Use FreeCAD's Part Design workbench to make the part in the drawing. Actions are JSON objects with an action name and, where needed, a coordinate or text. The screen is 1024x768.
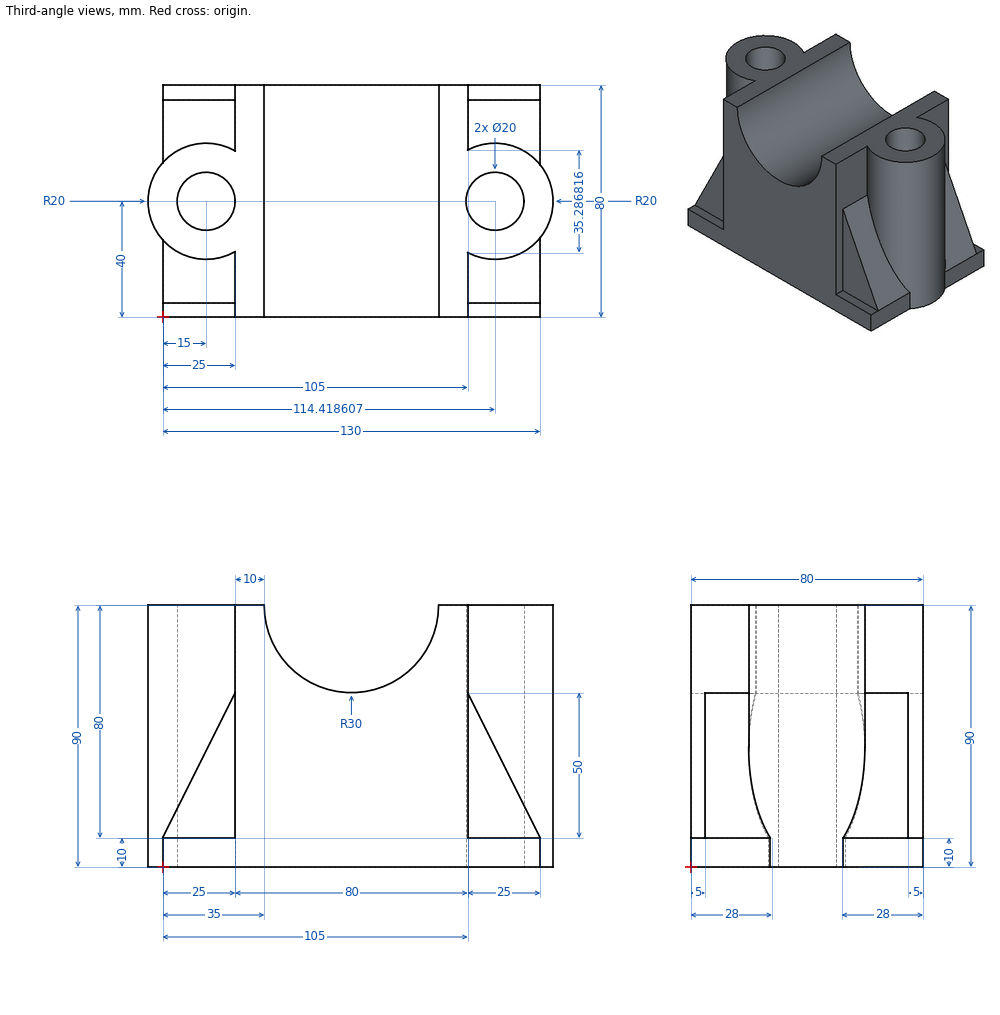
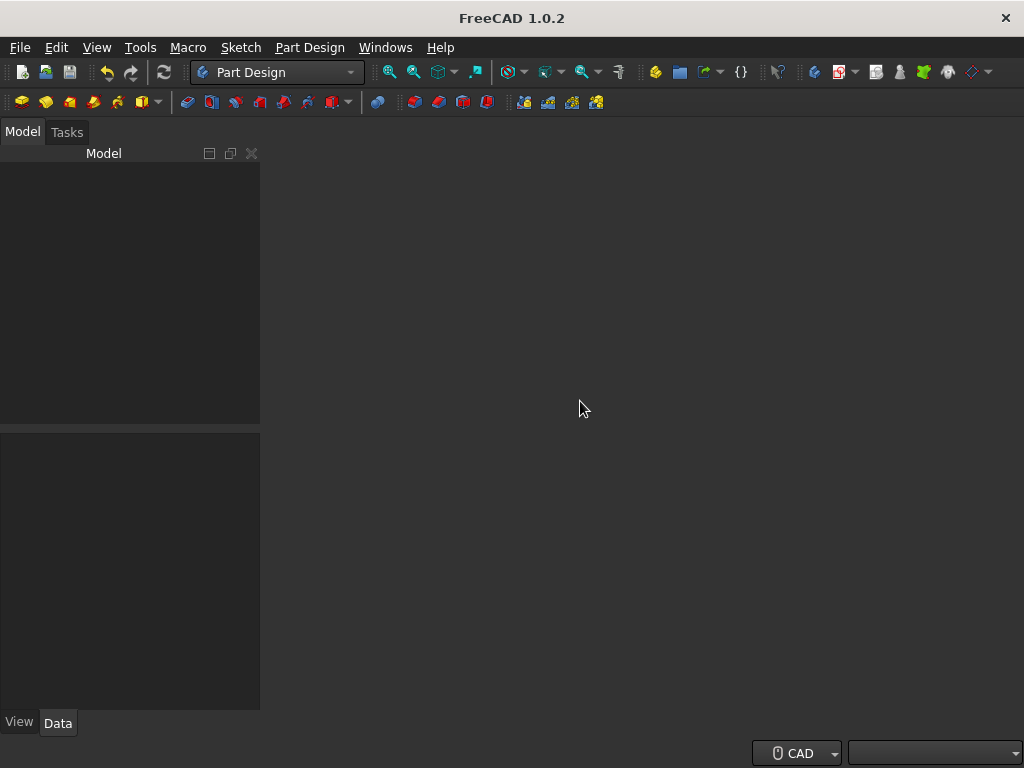
{"action": "left_click", "coordinate": [22, 72]}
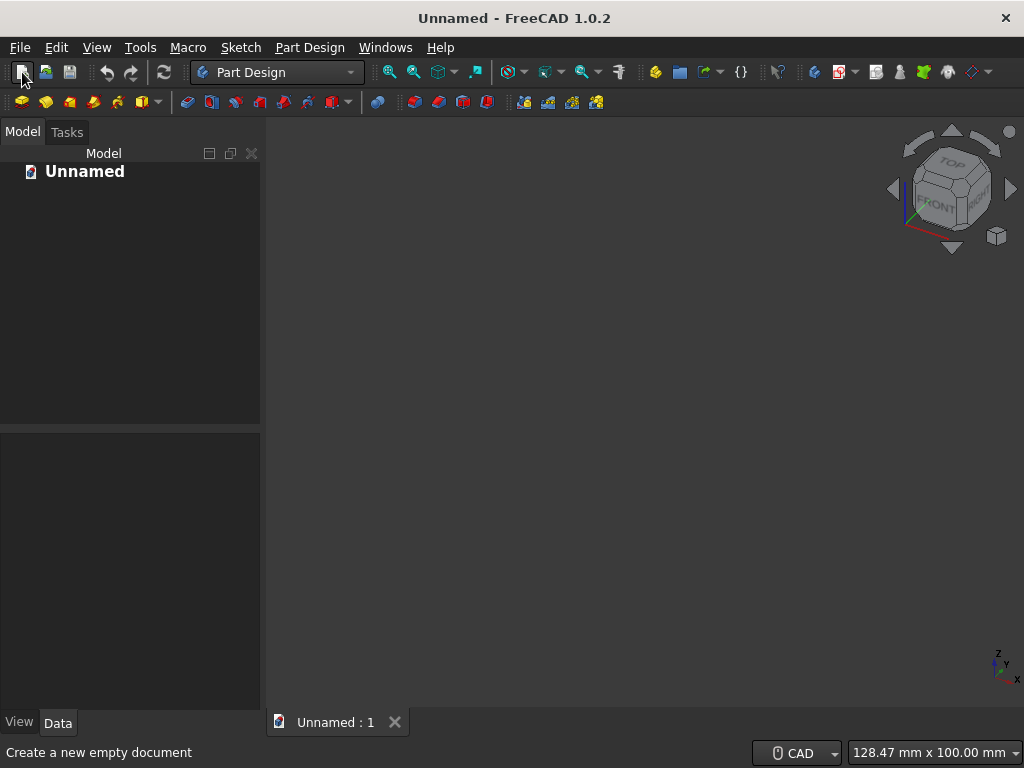
{"action": "left_click", "coordinate": [840, 72]}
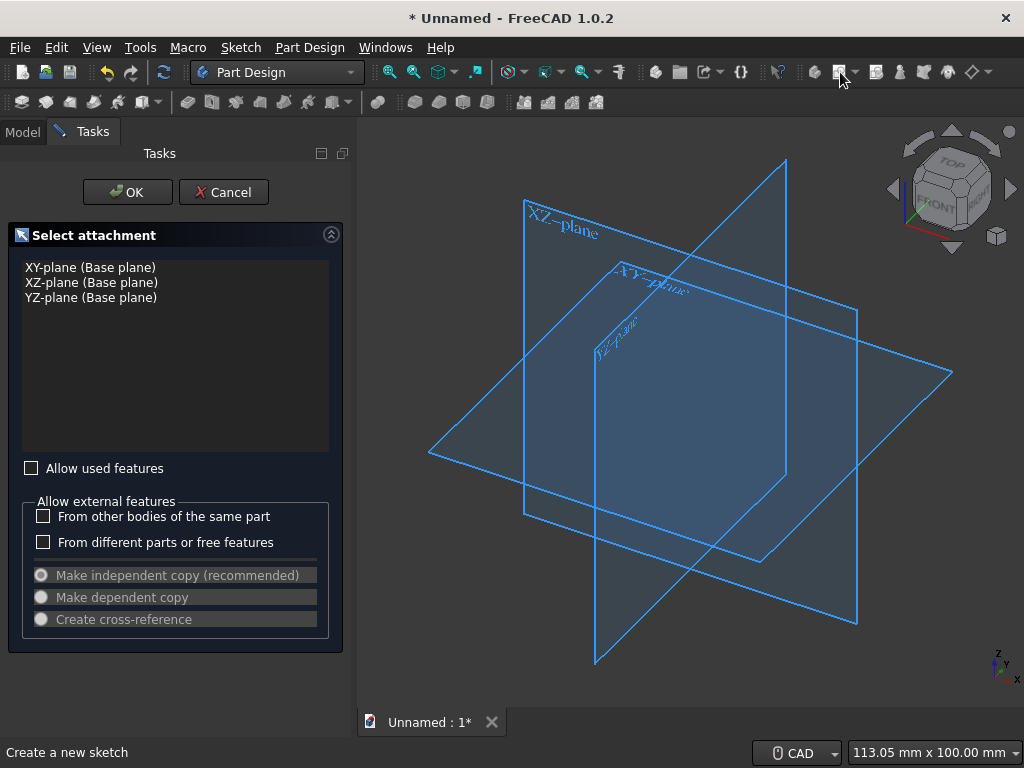
{"action": "left_click", "coordinate": [82, 268]}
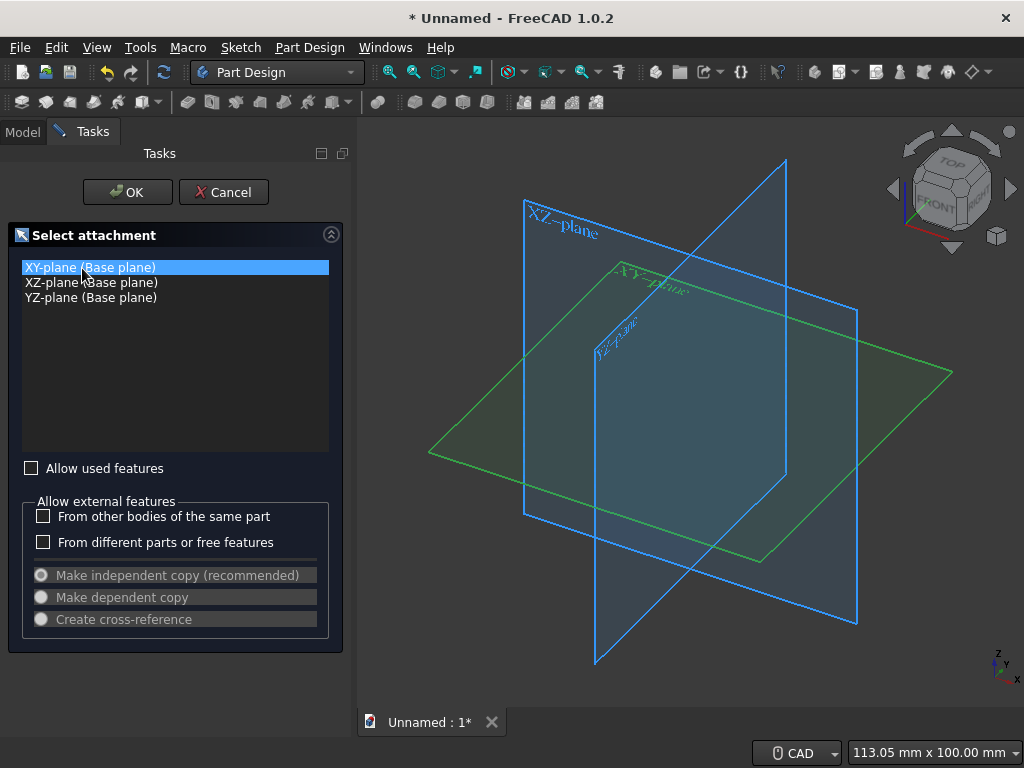
{"action": "left_click", "coordinate": [128, 192]}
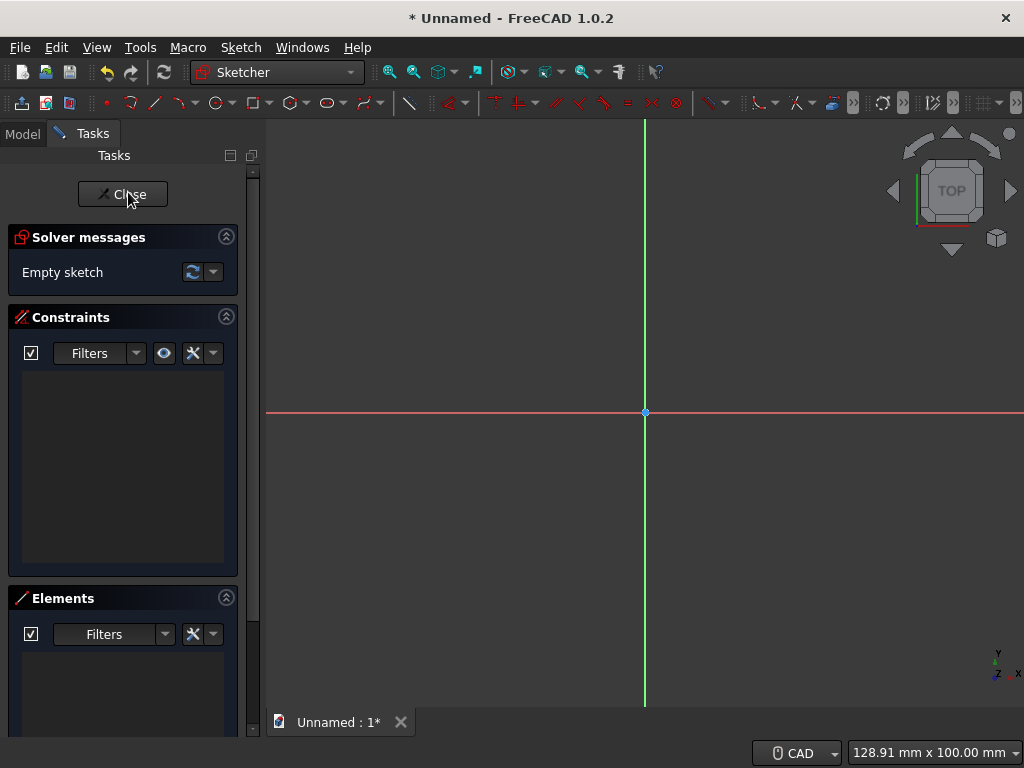
{"action": "scroll", "coordinate": [294, 605], "scroll_direction": "down", "scroll_amount": 4}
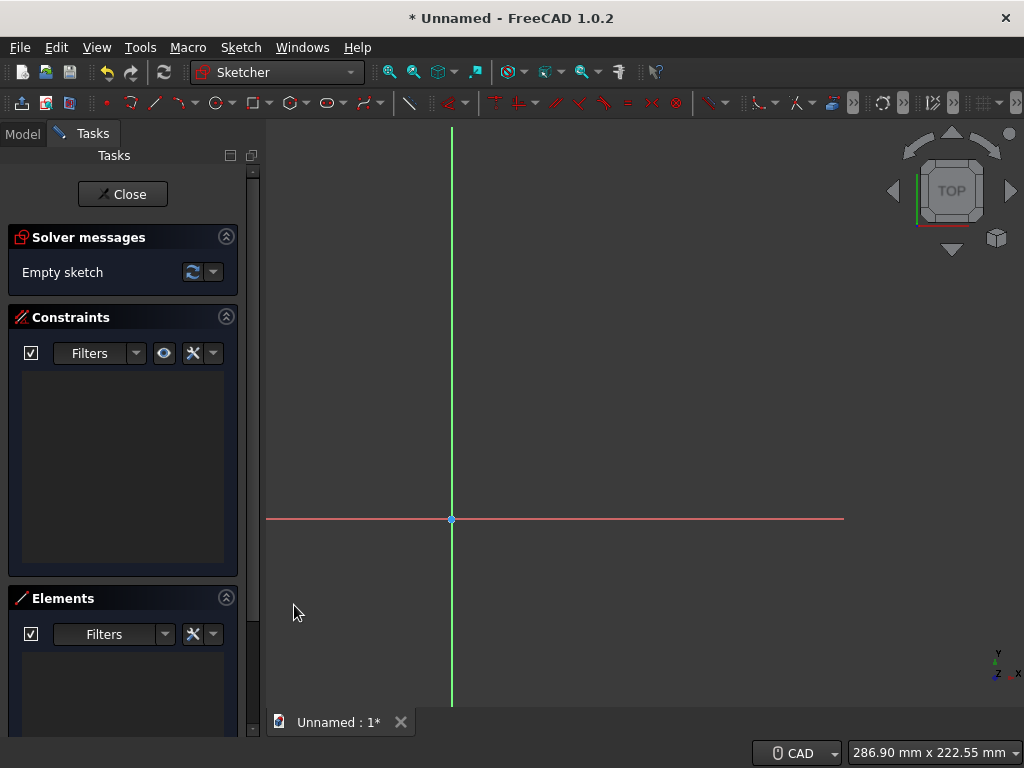
{"action": "left_click", "coordinate": [254, 104]}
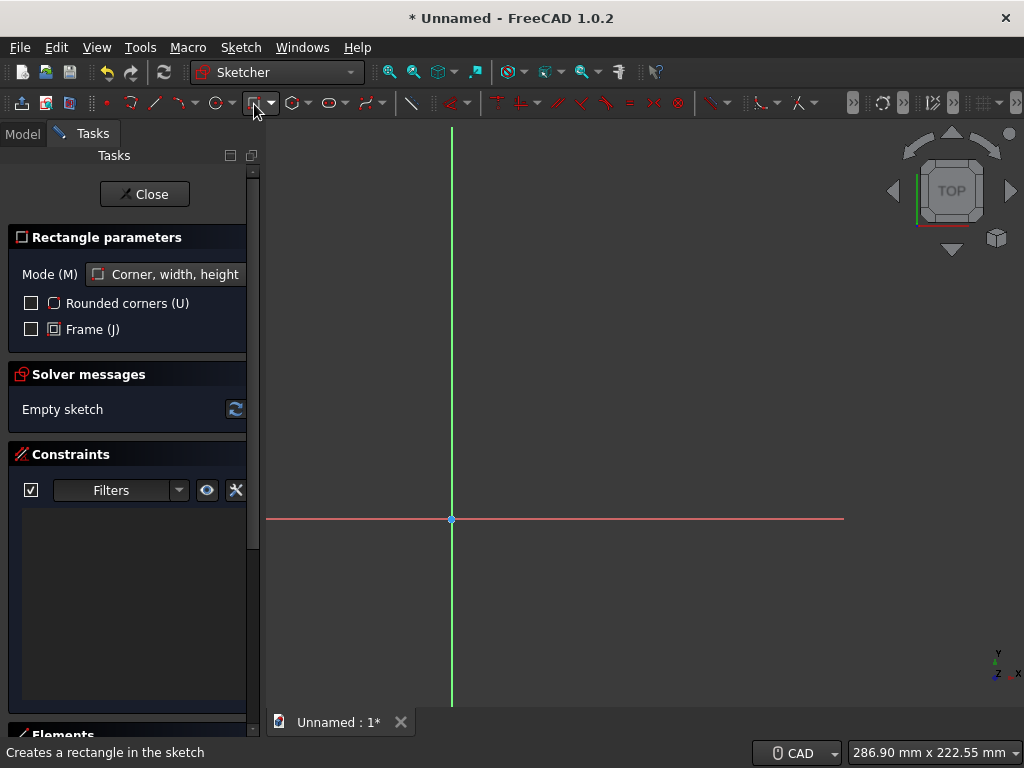
{"action": "left_click", "coordinate": [452, 519]}
{"action": "left_click", "coordinate": [795, 308]}
{"action": "key", "text": "Escape"}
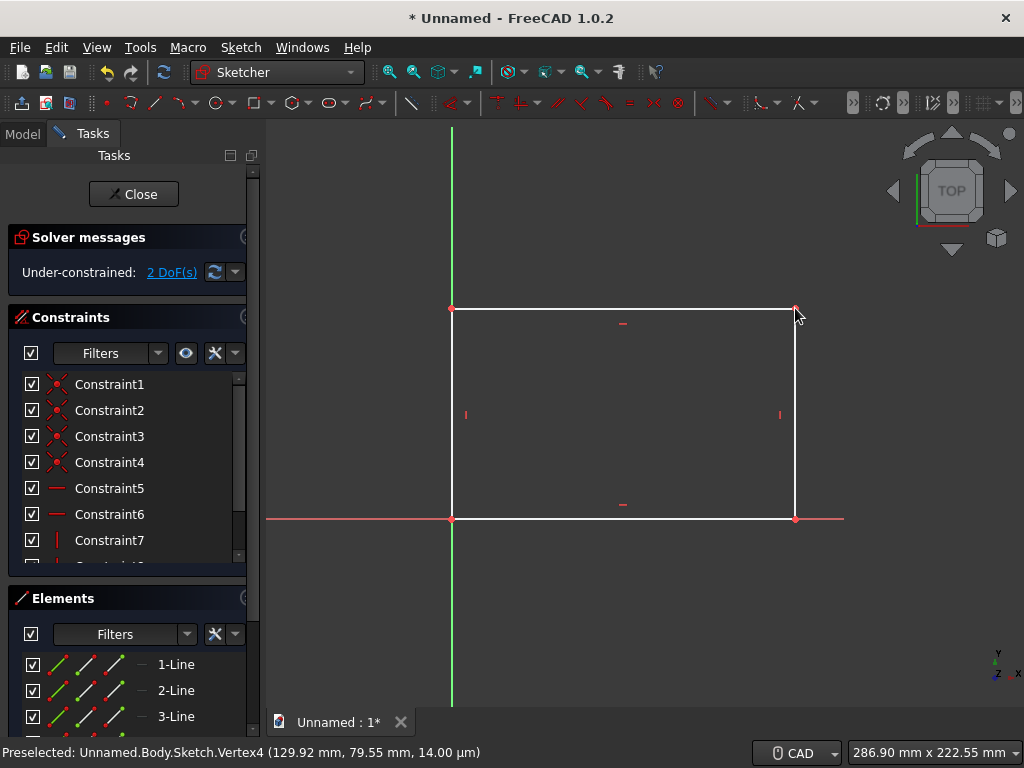
{"action": "left_click", "coordinate": [450, 104]}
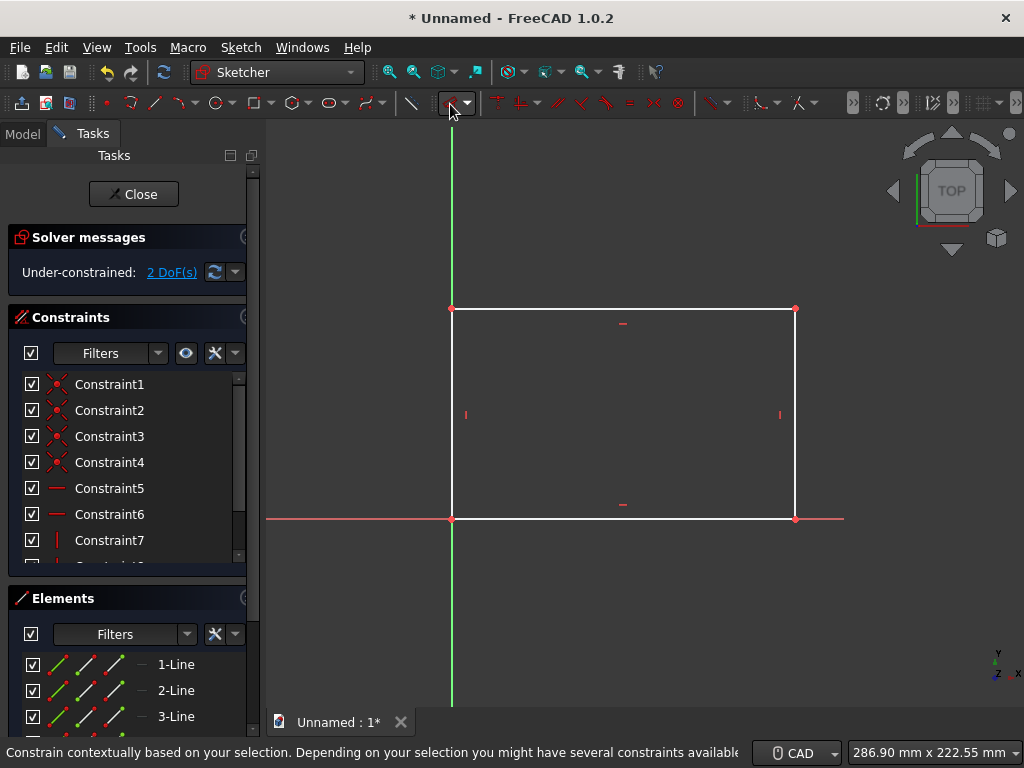
{"action": "left_click", "coordinate": [795, 456]}
{"action": "left_click", "coordinate": [829, 414]}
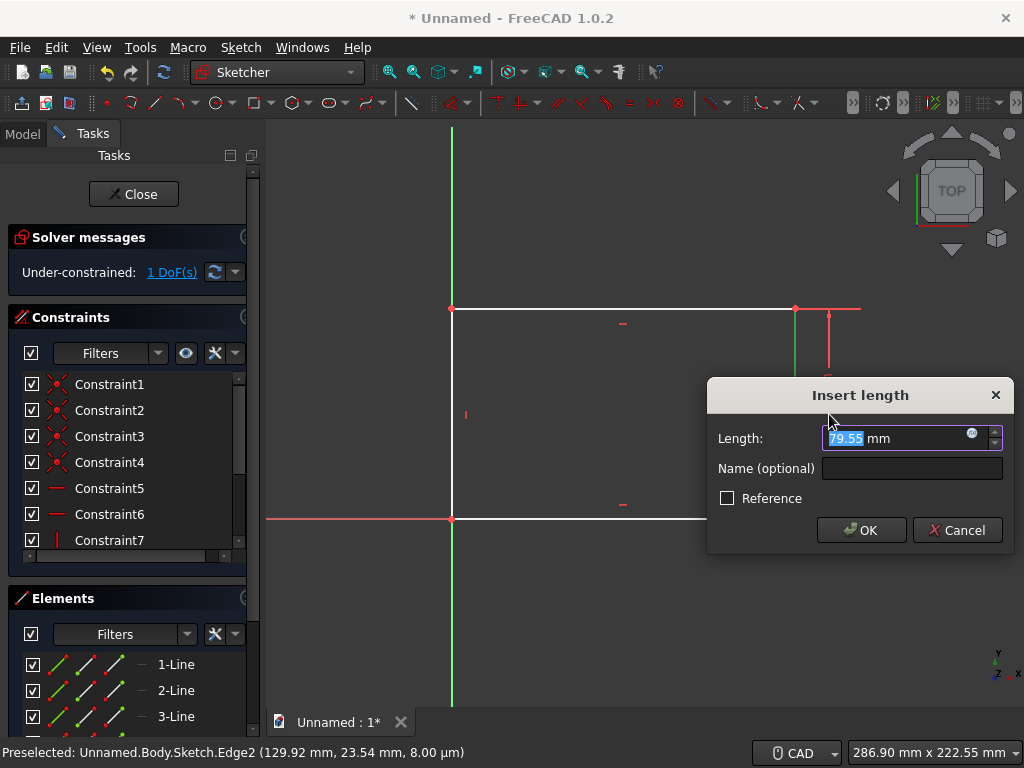
{"action": "type", "text": "80"}
{"action": "key", "text": "Return"}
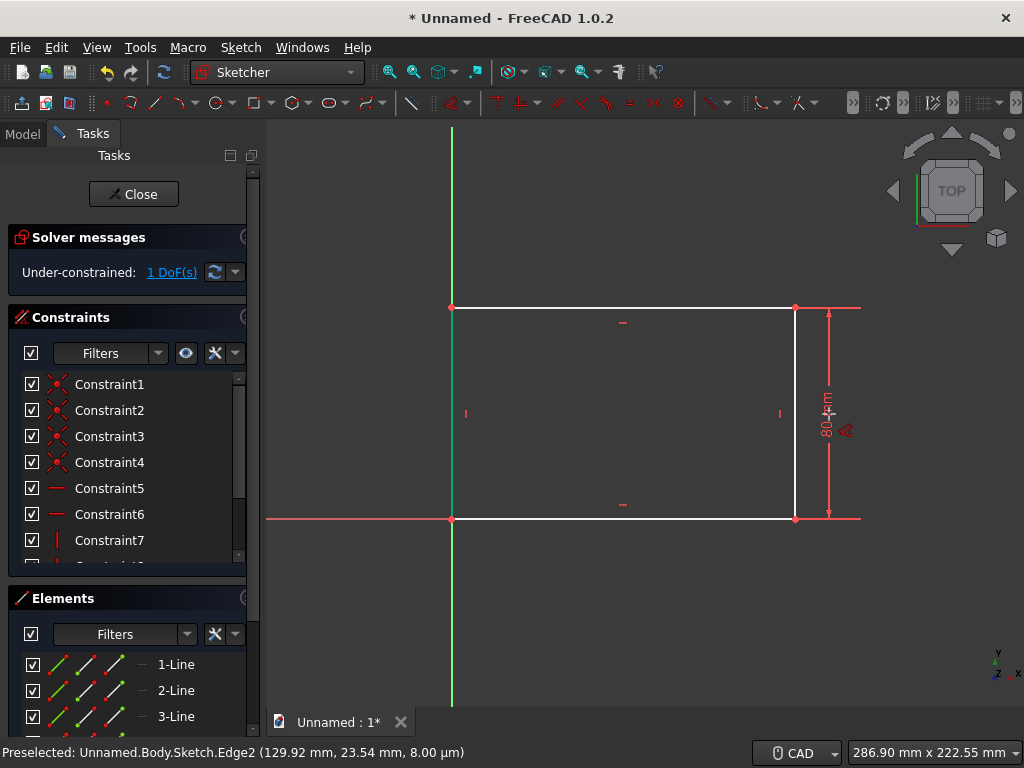
{"action": "left_click", "coordinate": [555, 519]}
{"action": "left_click", "coordinate": [623, 553]}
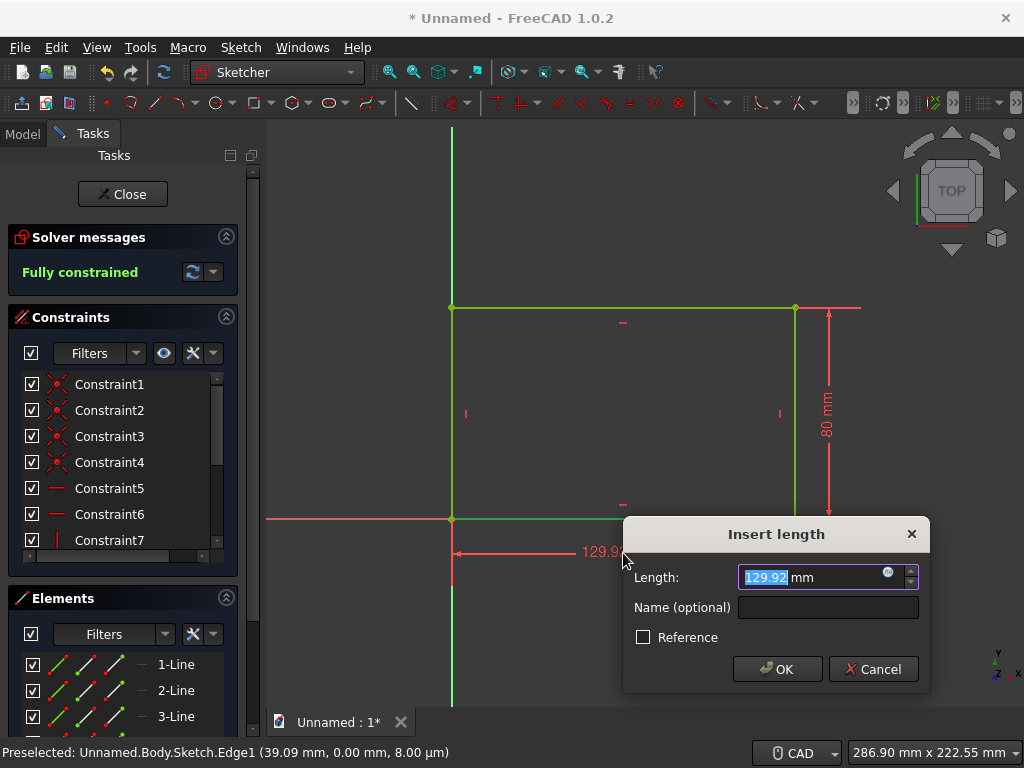
{"action": "type", "text": "130"}
{"action": "key", "text": "Return"}
{"action": "key", "text": "Escape"}